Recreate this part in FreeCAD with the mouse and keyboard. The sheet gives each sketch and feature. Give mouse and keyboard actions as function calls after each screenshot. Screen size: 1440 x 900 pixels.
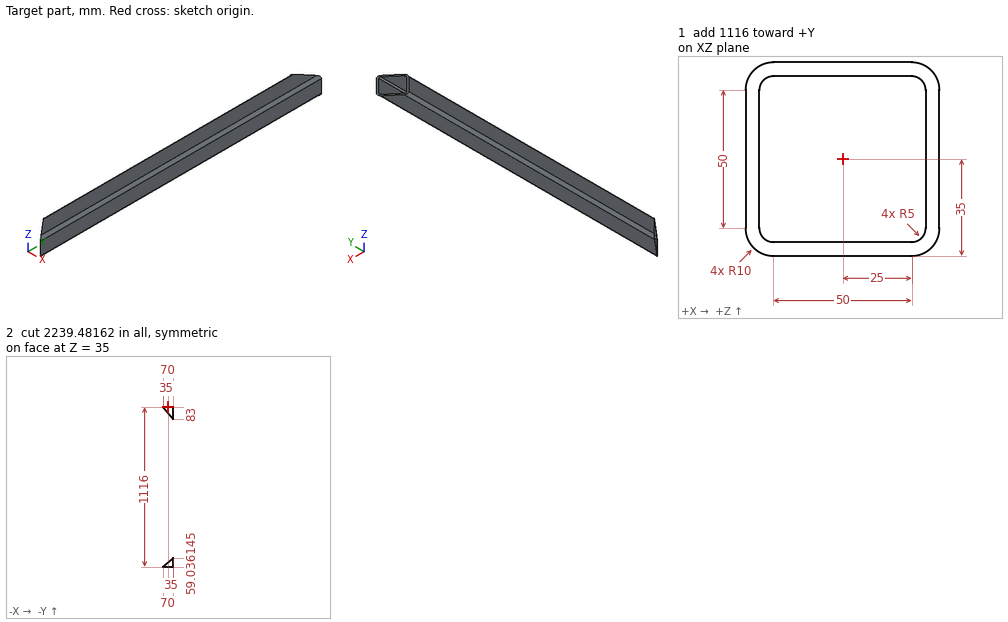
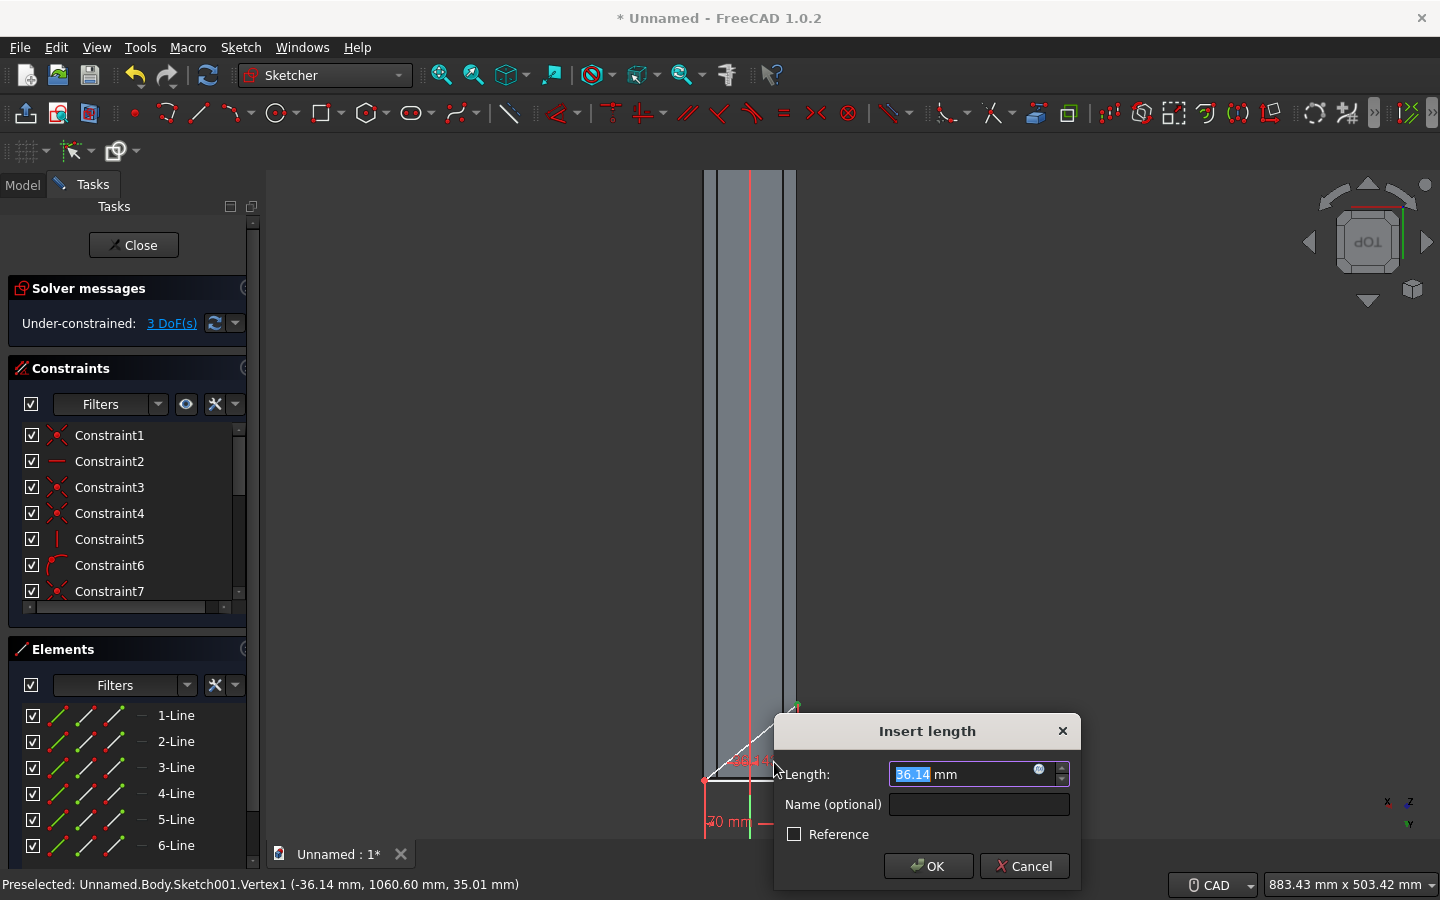
text(35)
key(Return)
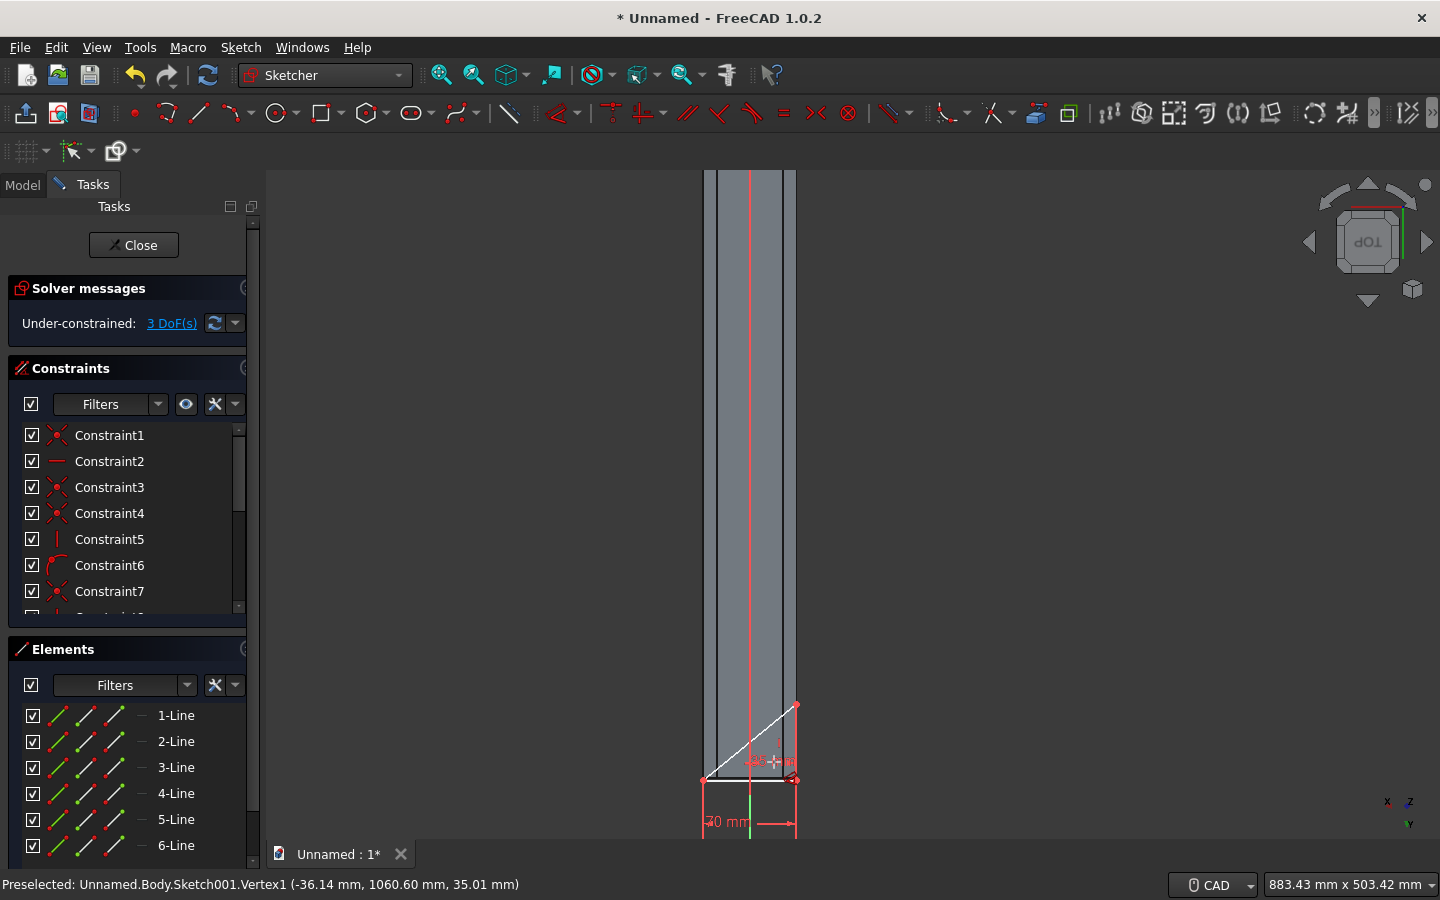
scroll(799, 706, down, 6)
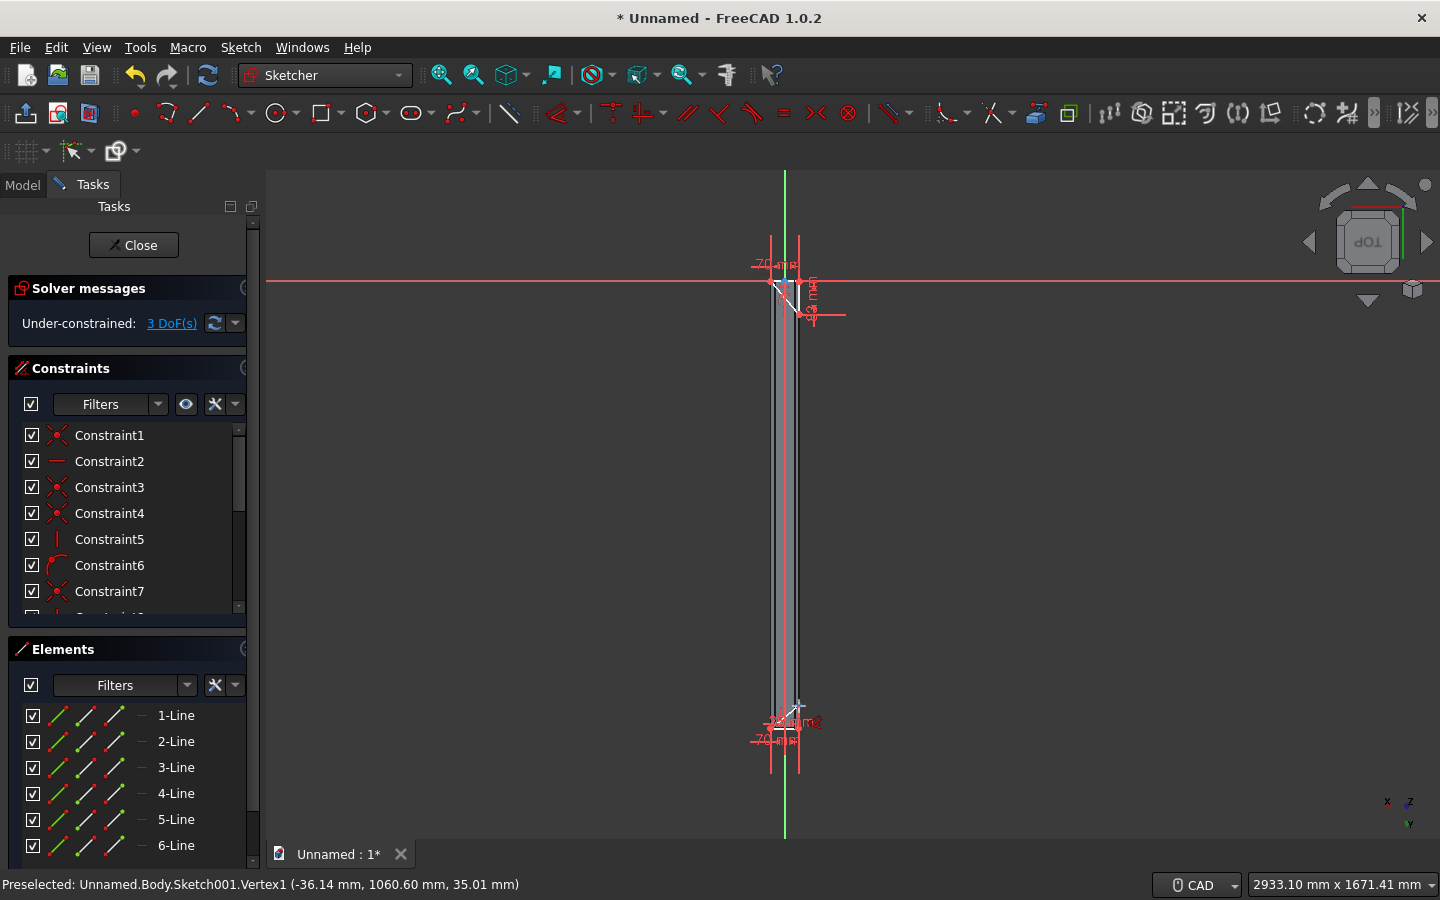
scroll(771, 281, up, 6)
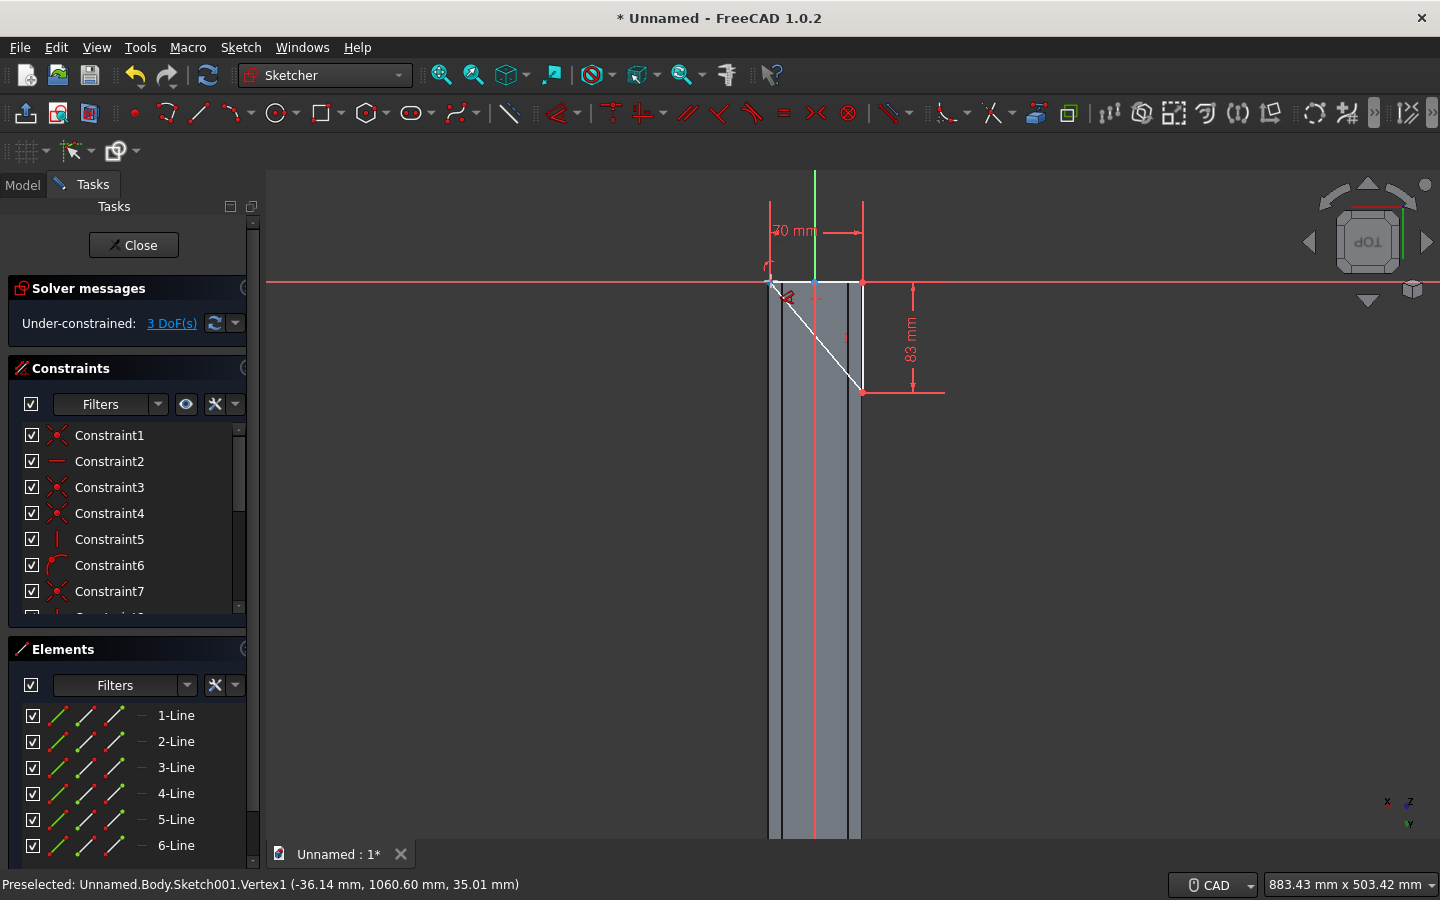
click(770, 282)
click(777, 316)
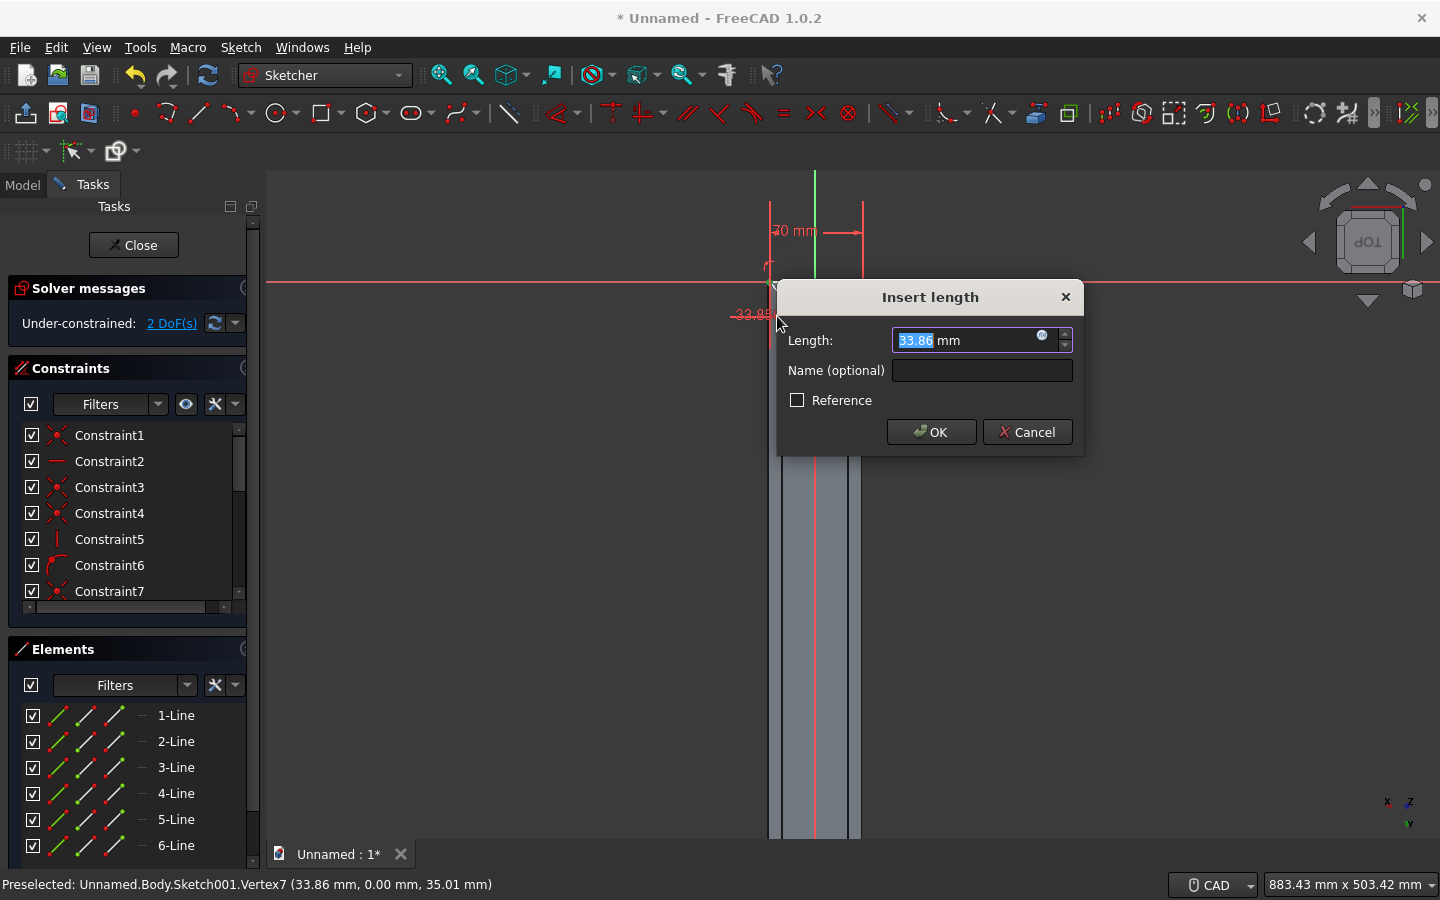
text(35)
key(Return)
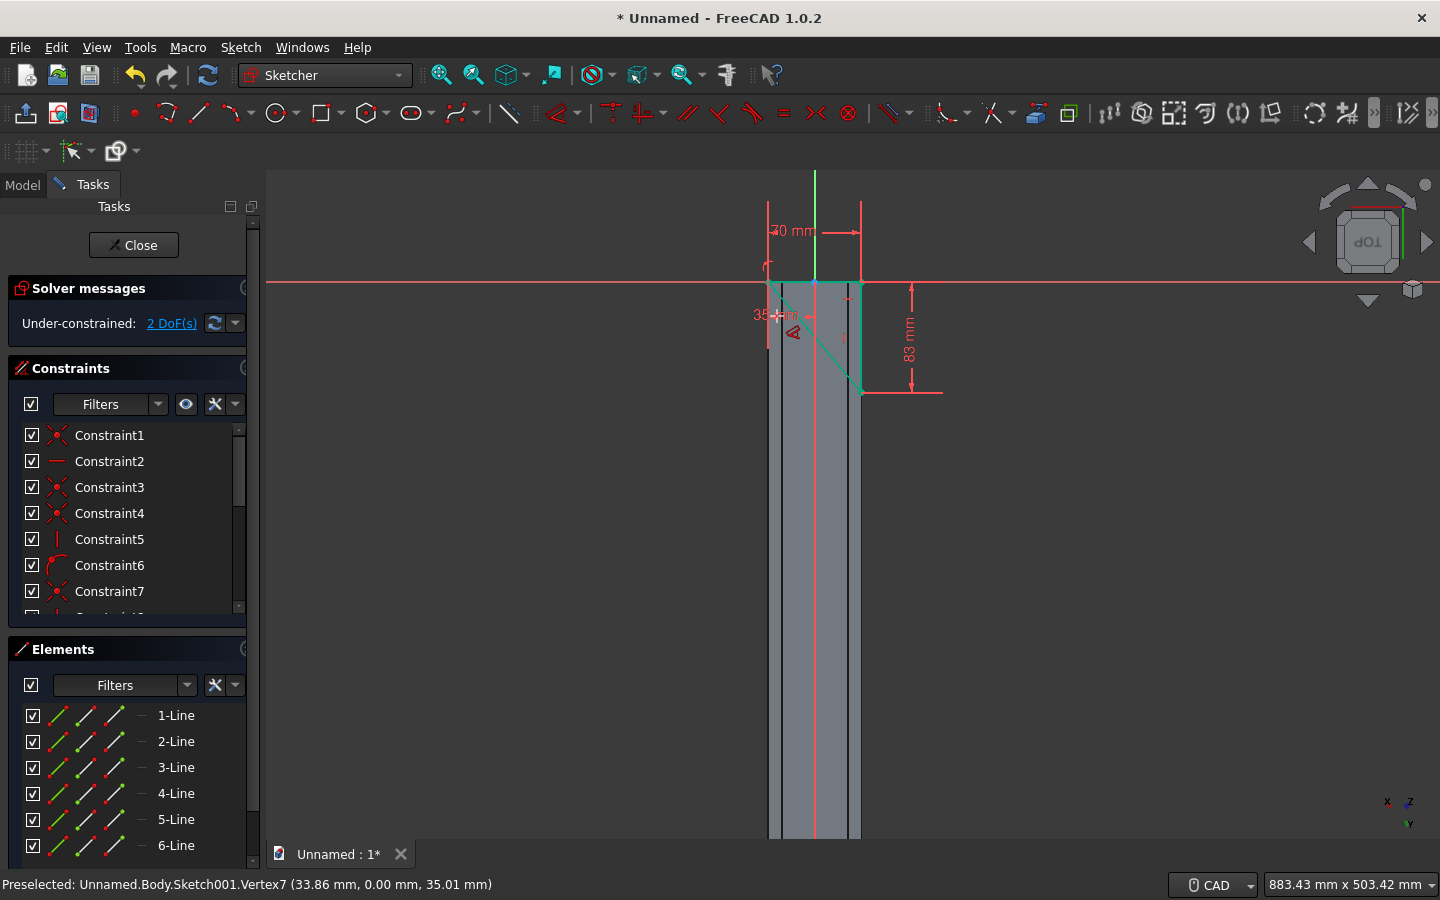
scroll(771, 281, down, 6)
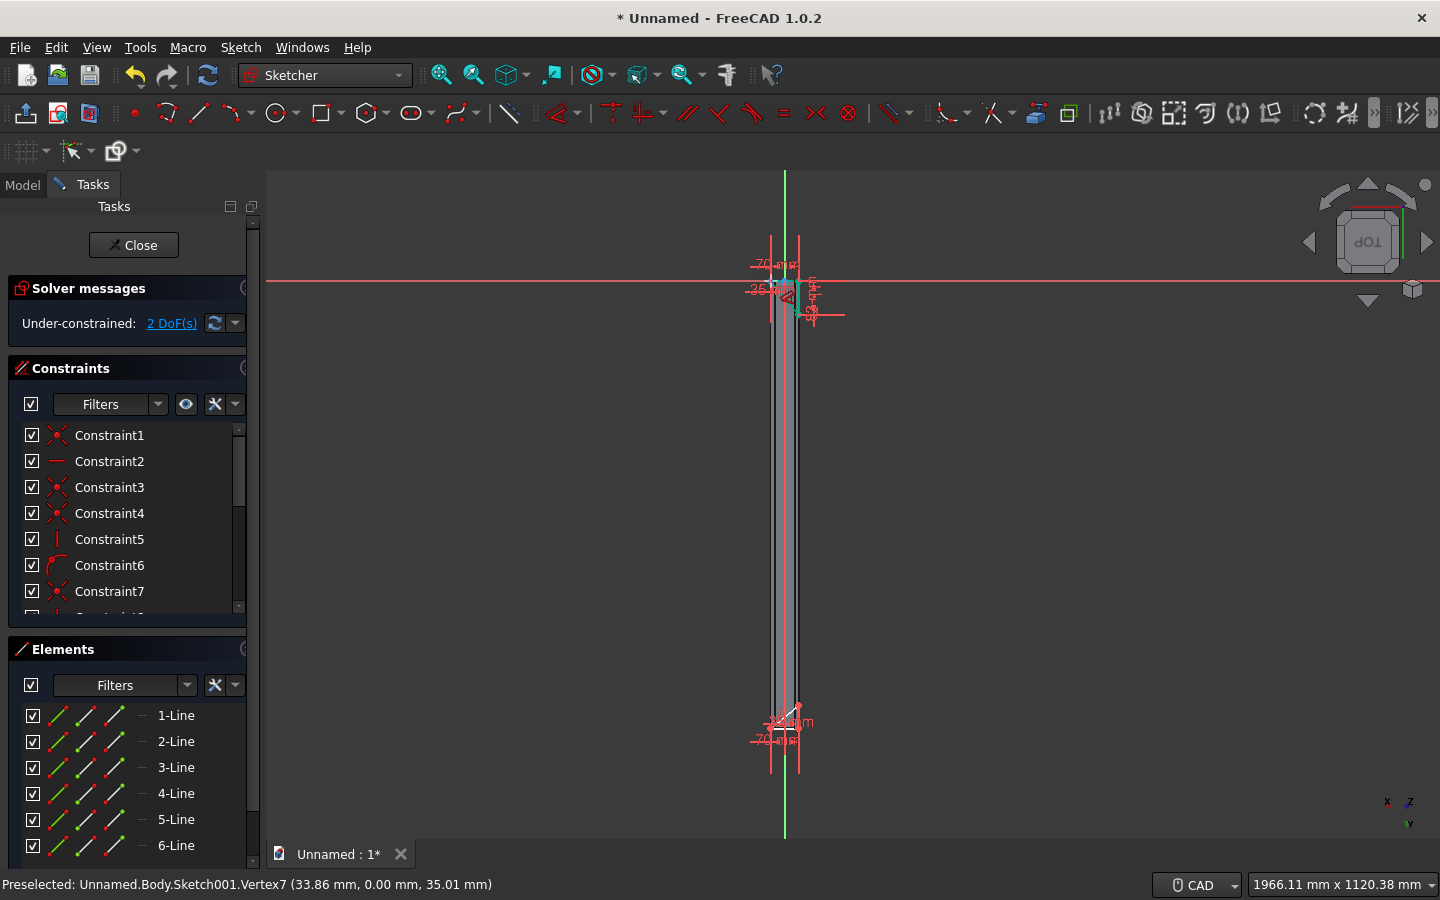
click(771, 729)
click(737, 505)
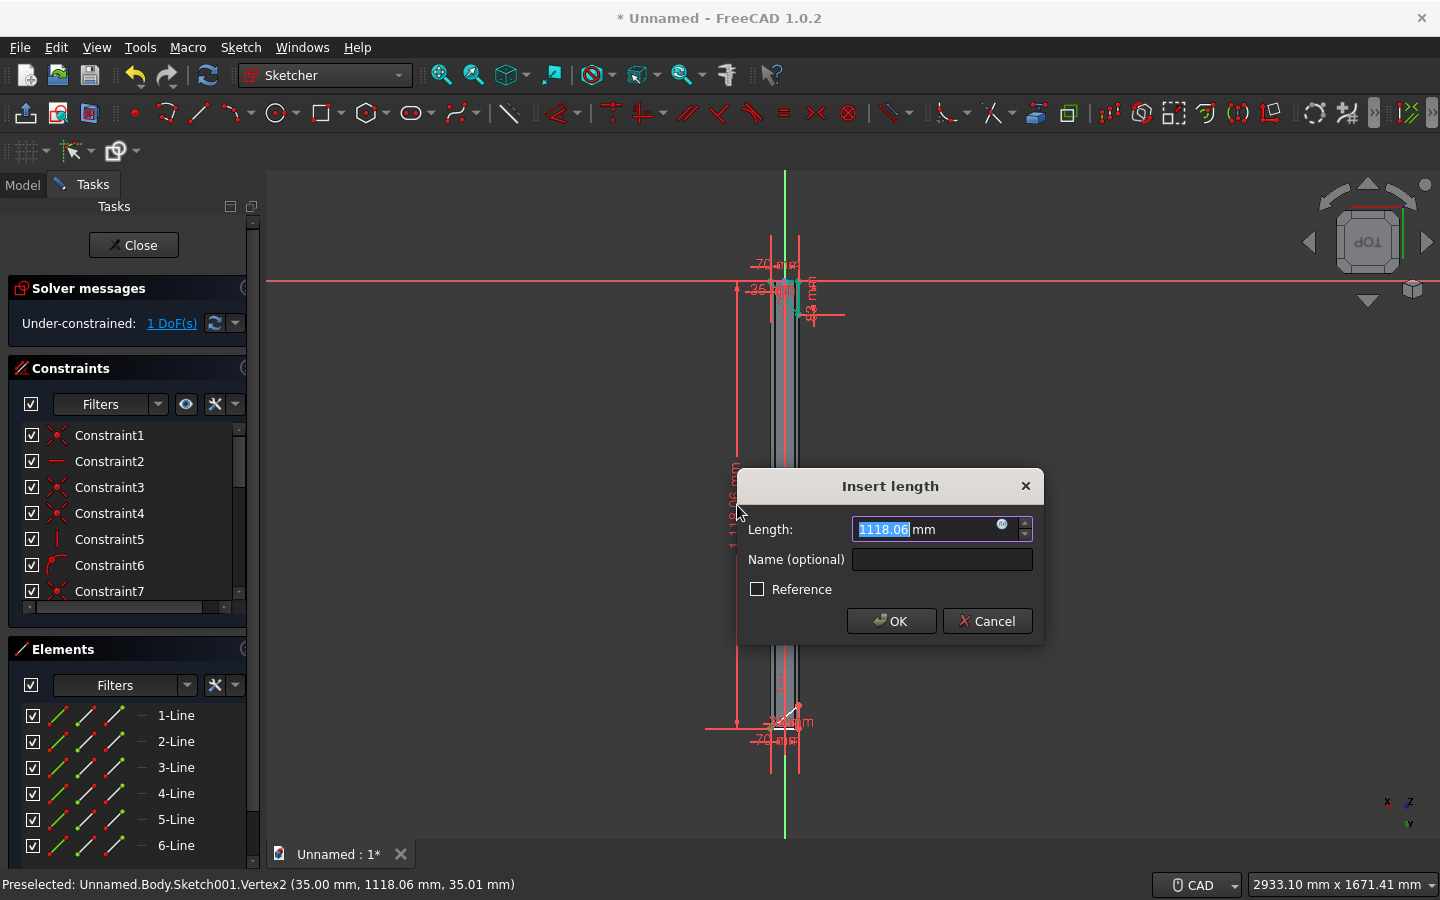
text(1116)
key(Return)